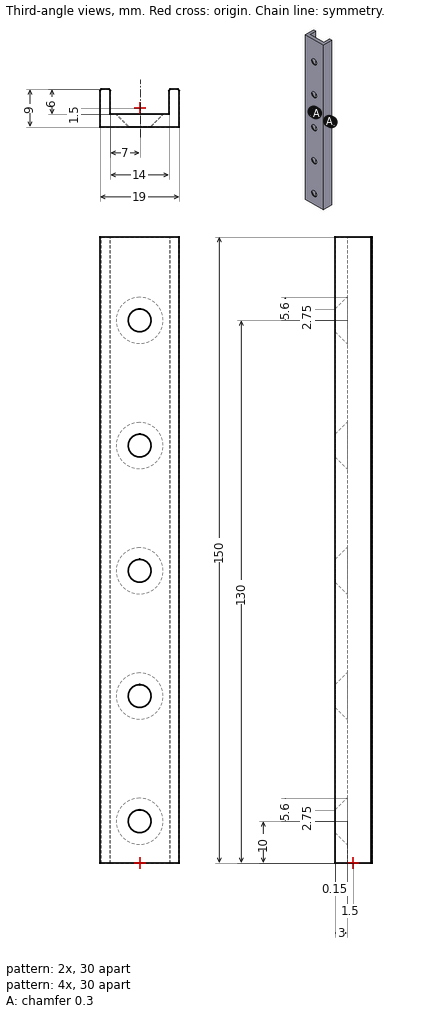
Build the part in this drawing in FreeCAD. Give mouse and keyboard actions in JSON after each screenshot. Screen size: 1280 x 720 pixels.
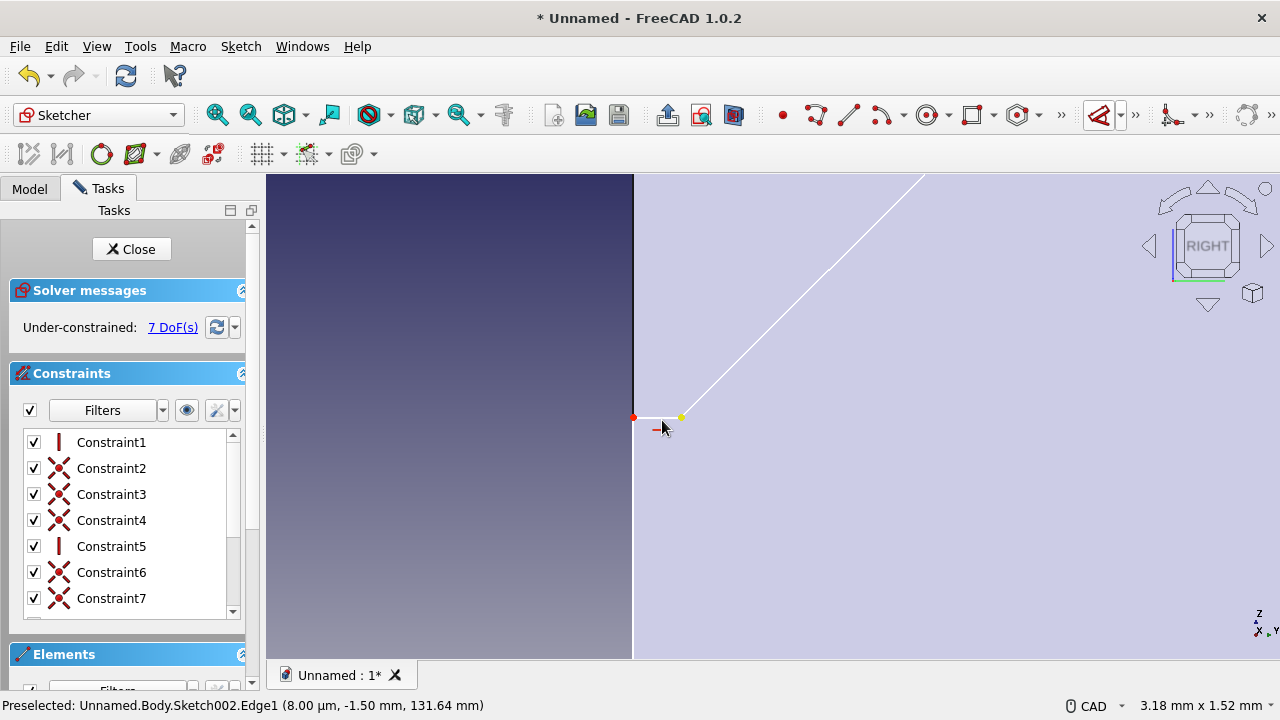
{"action": "left_click", "coordinate": [657, 418]}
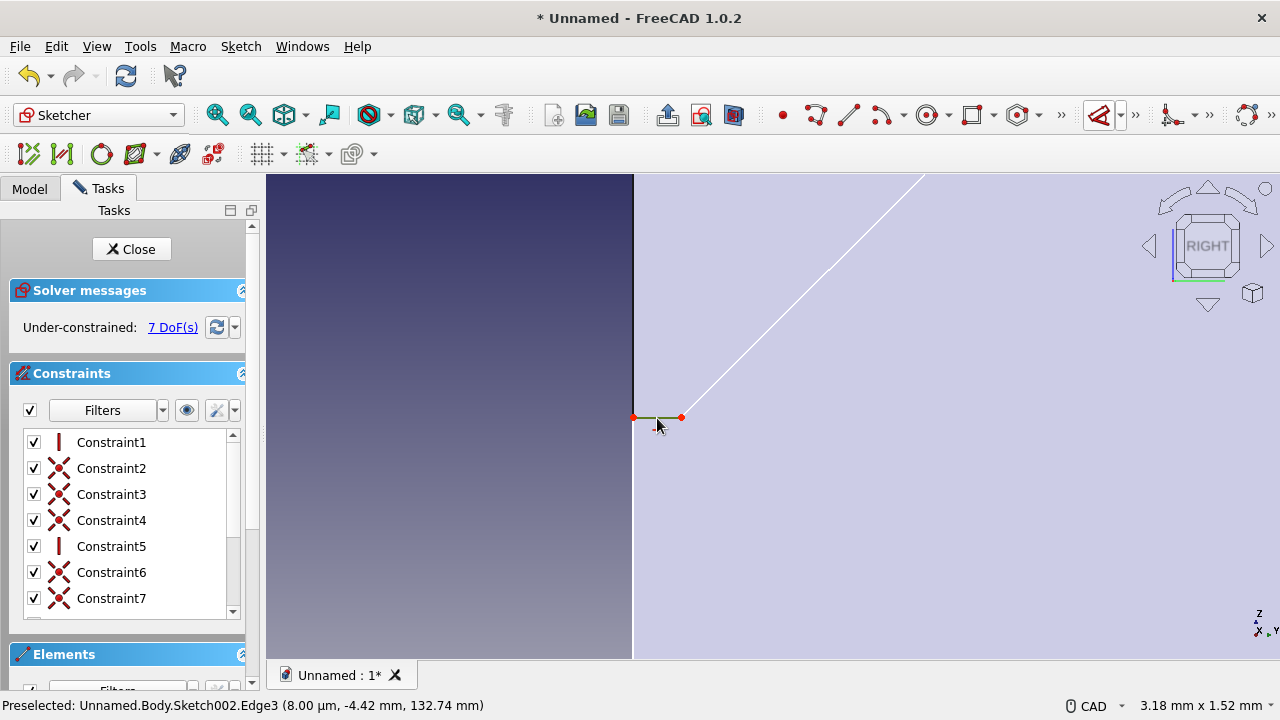
{"action": "left_click", "coordinate": [1120, 116]}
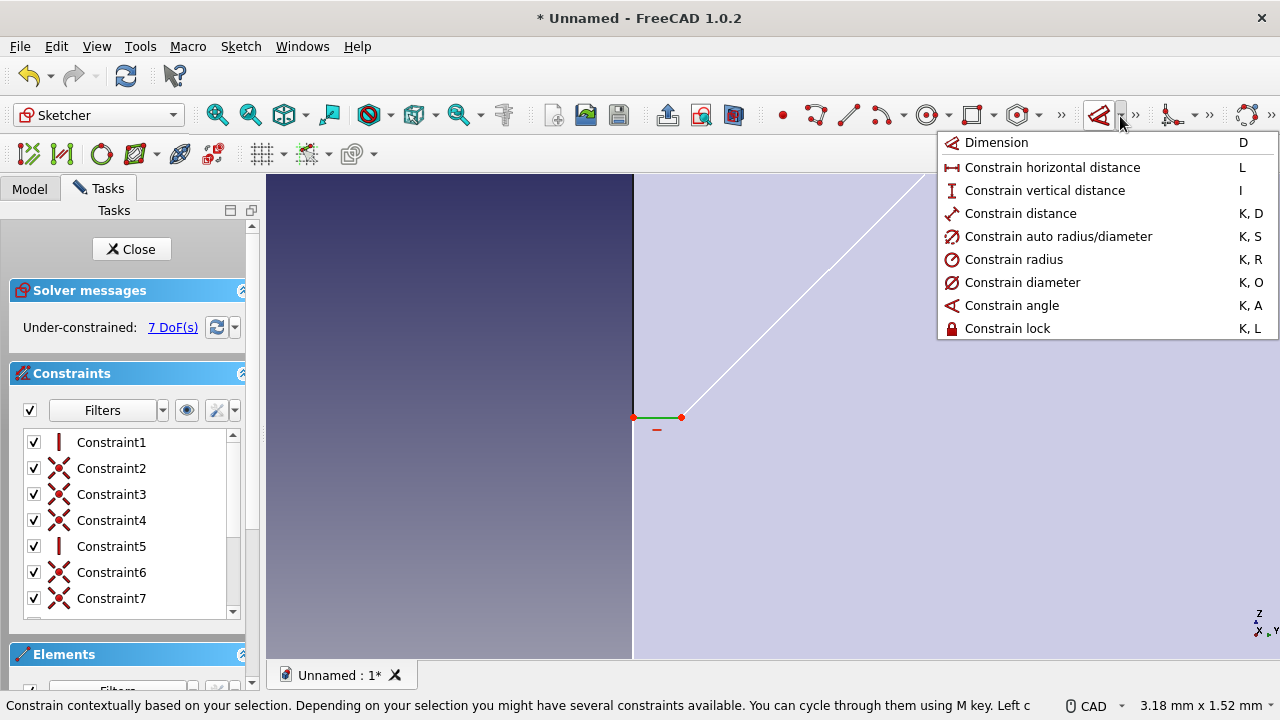
{"action": "left_click", "coordinate": [1108, 168]}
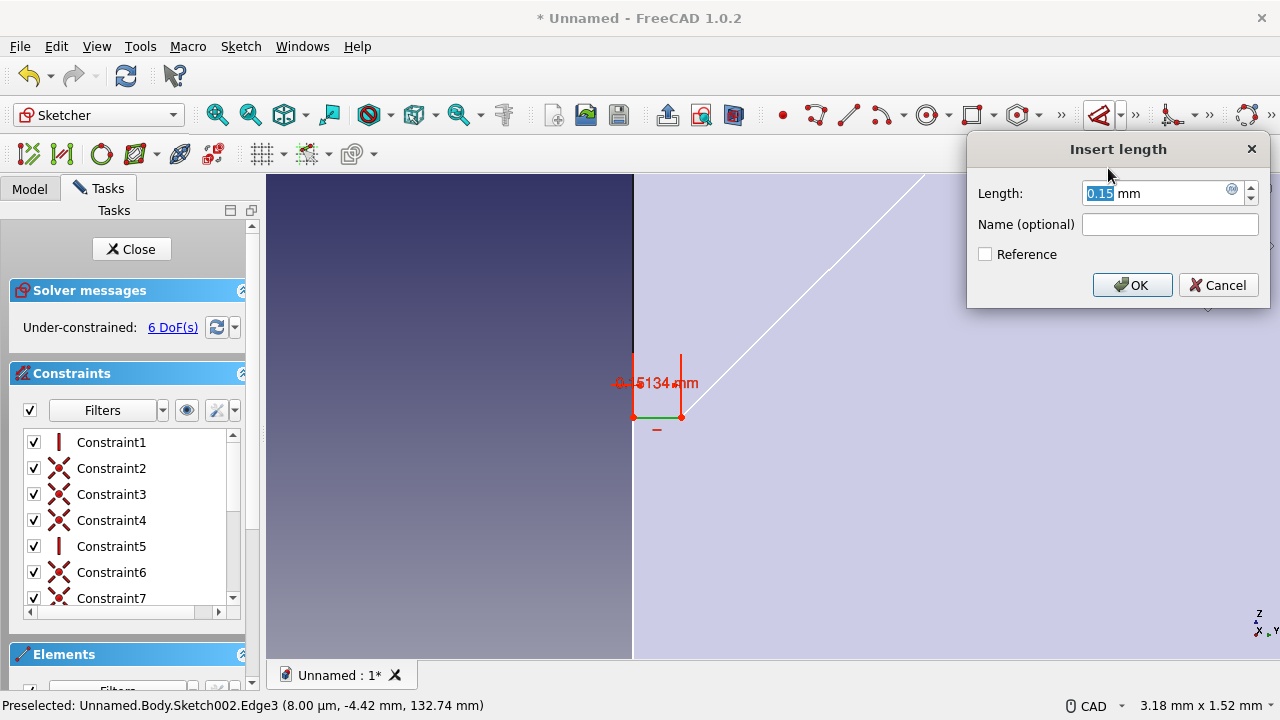
{"action": "type", "text": "0.15"}
{"action": "key", "text": "Return"}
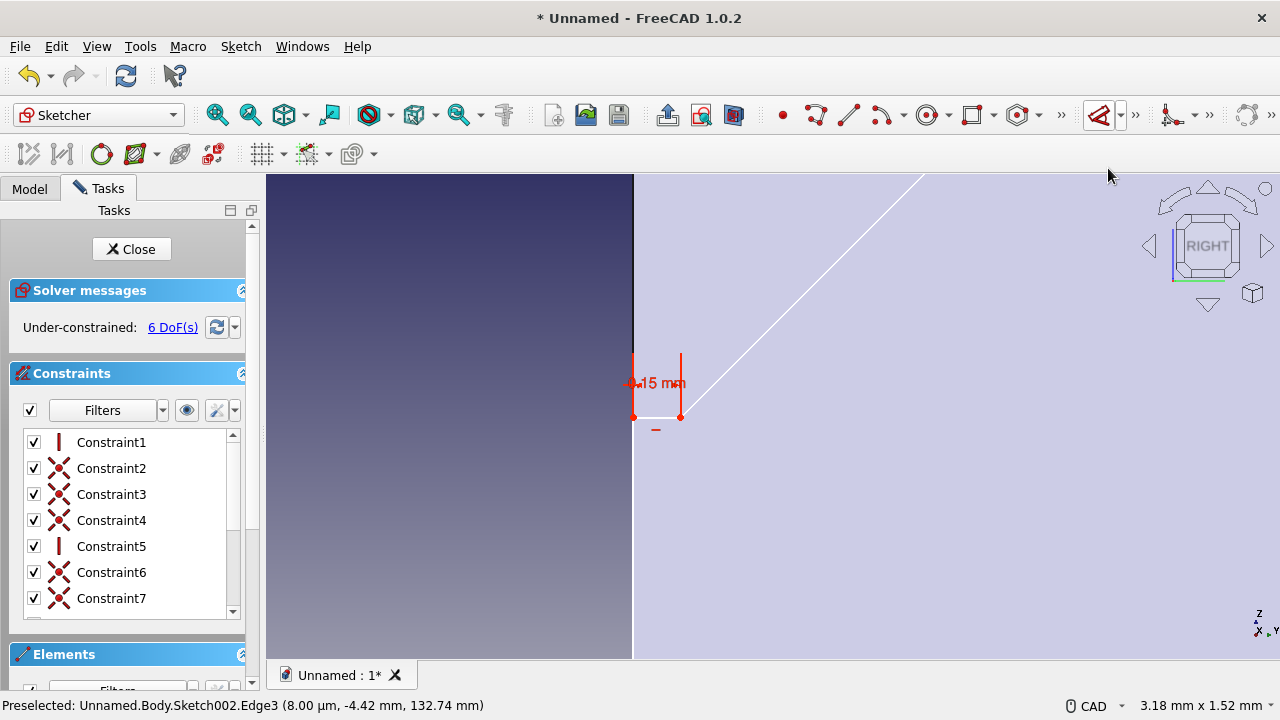
{"action": "scroll", "coordinate": [662, 420], "scroll_direction": "down", "scroll_amount": 9}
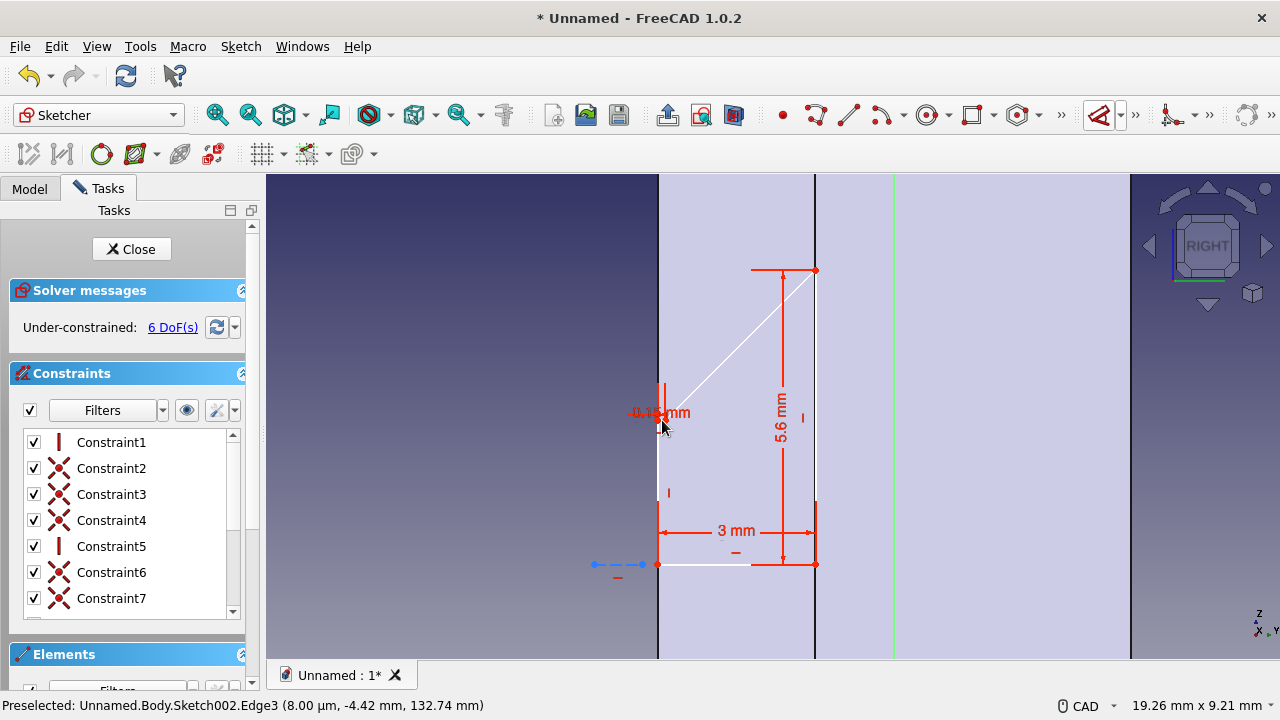
{"action": "left_click", "coordinate": [658, 449]}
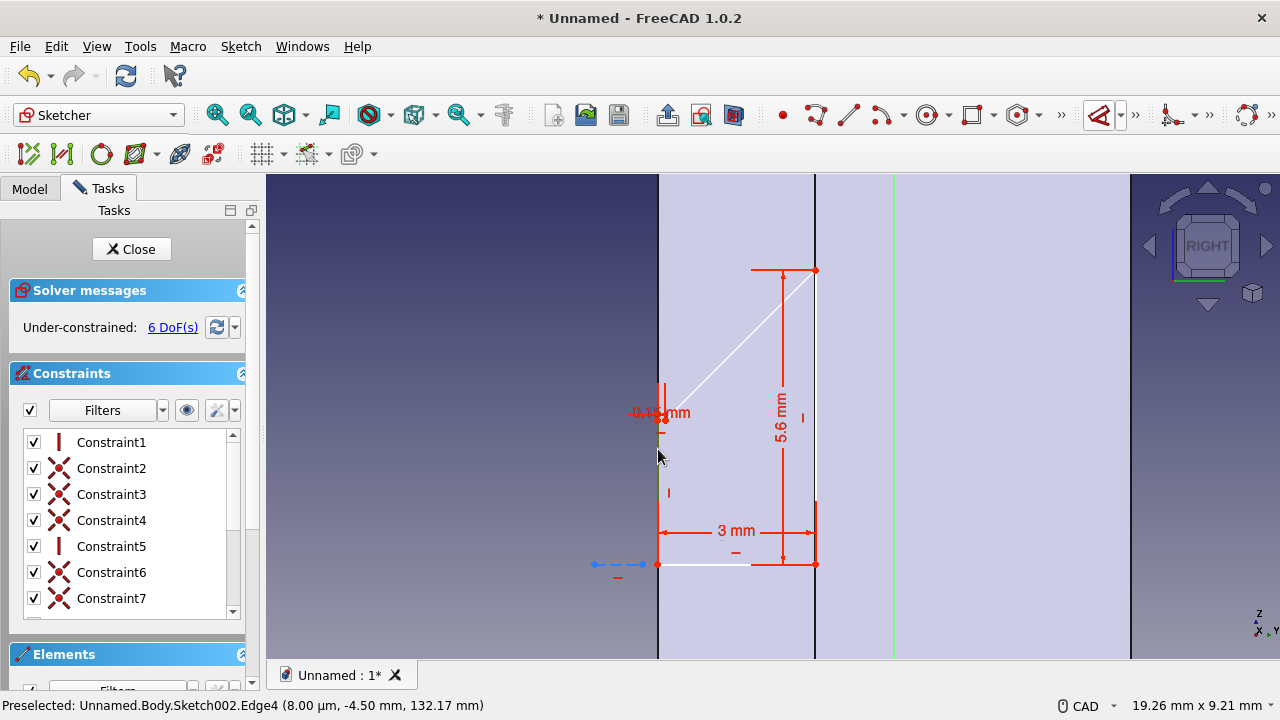
{"action": "left_click", "coordinate": [1120, 116]}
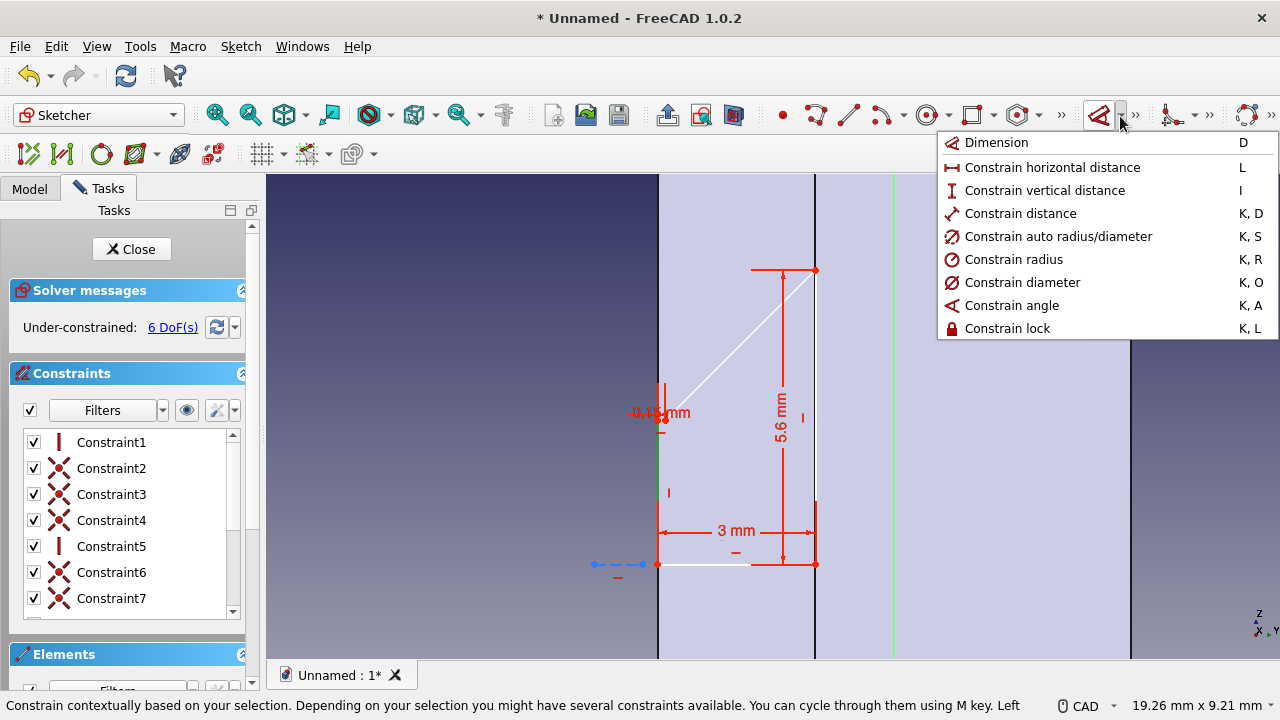
{"action": "left_click", "coordinate": [1108, 190]}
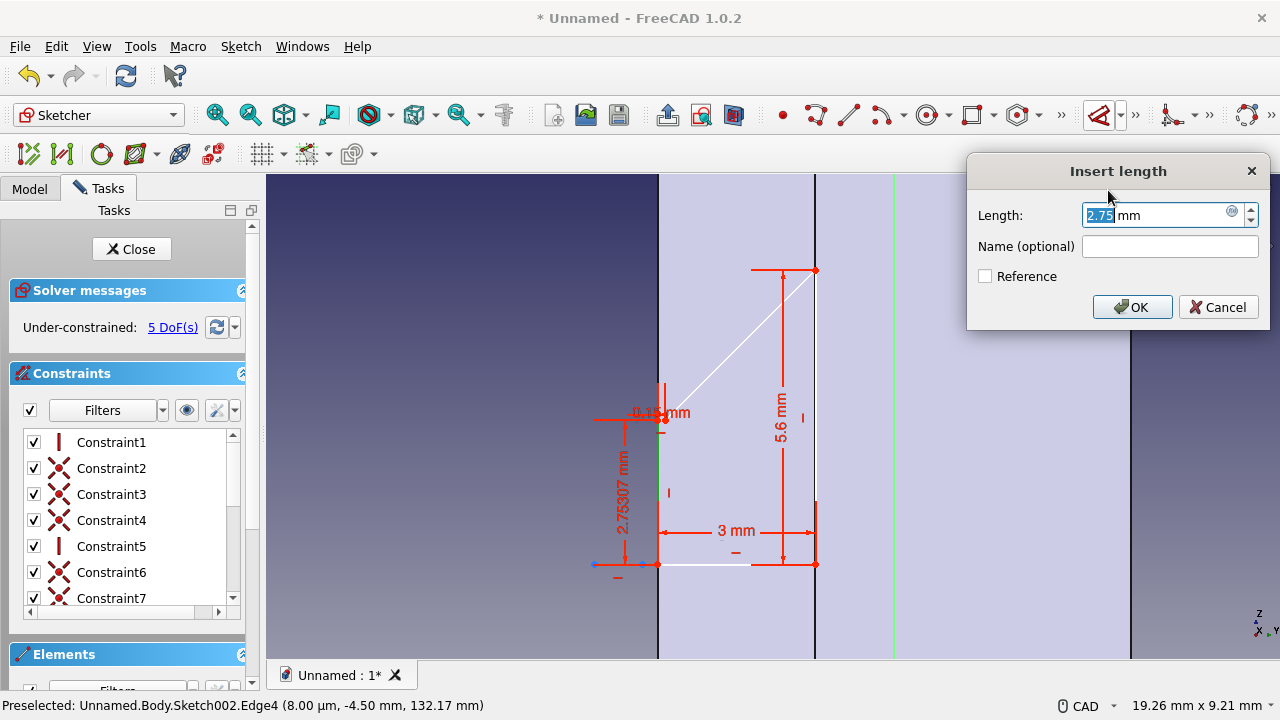
{"action": "type", "text": "2.75"}
{"action": "key", "text": "Return"}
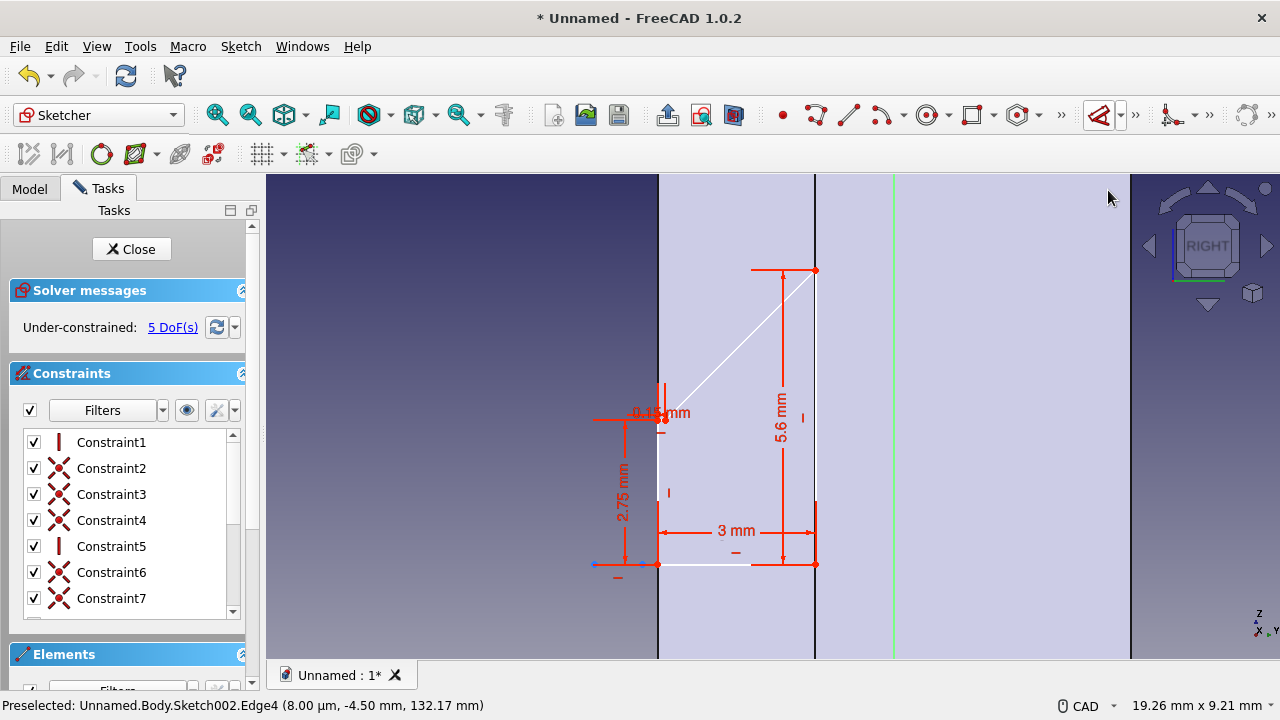
{"action": "left_click", "coordinate": [816, 565]}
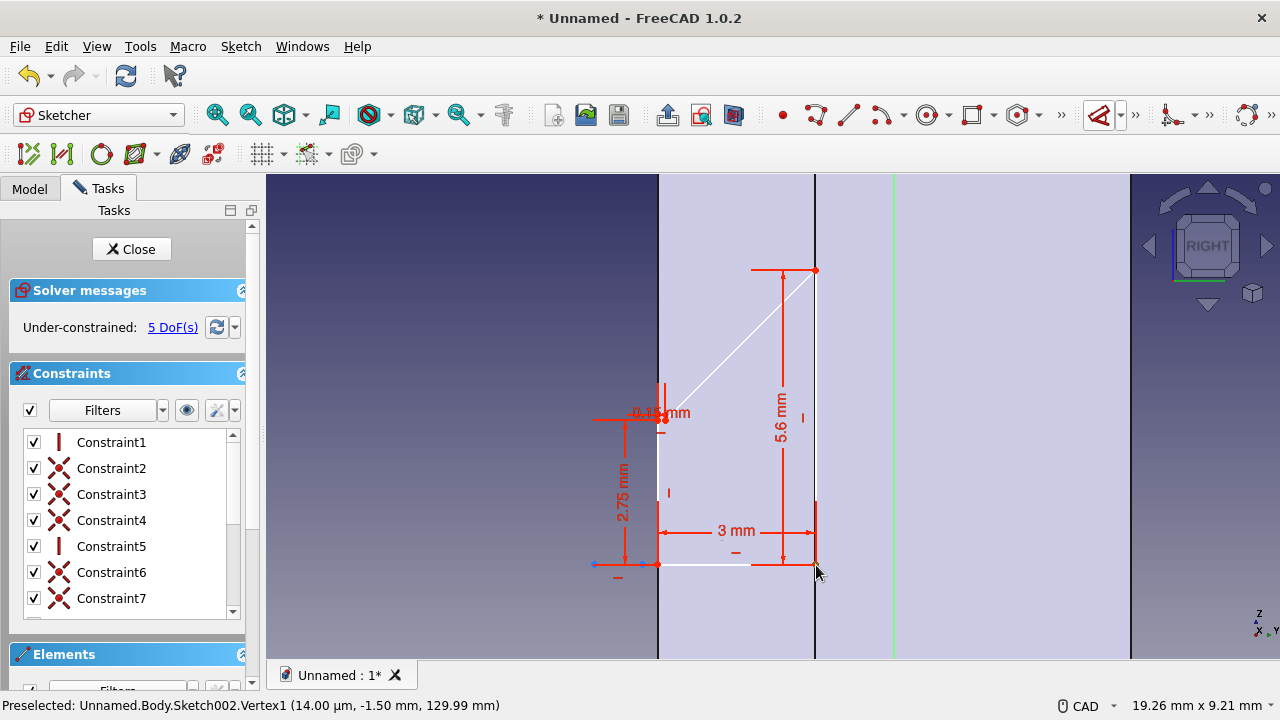
{"action": "key", "text": "l"}